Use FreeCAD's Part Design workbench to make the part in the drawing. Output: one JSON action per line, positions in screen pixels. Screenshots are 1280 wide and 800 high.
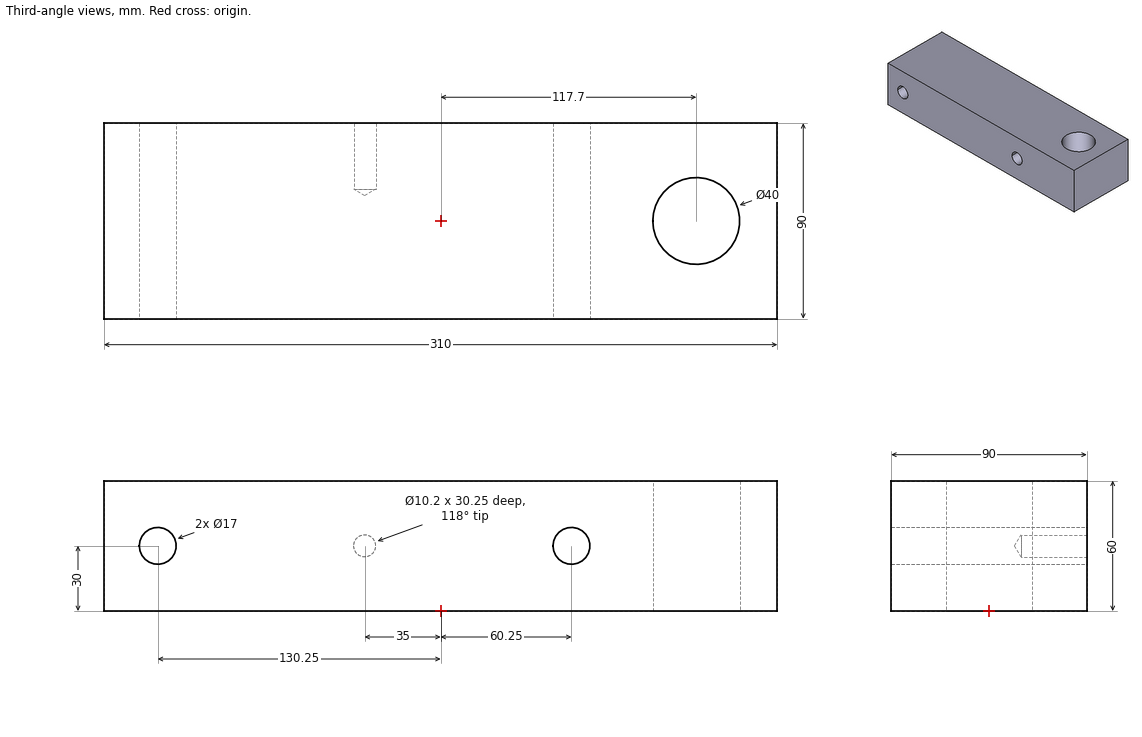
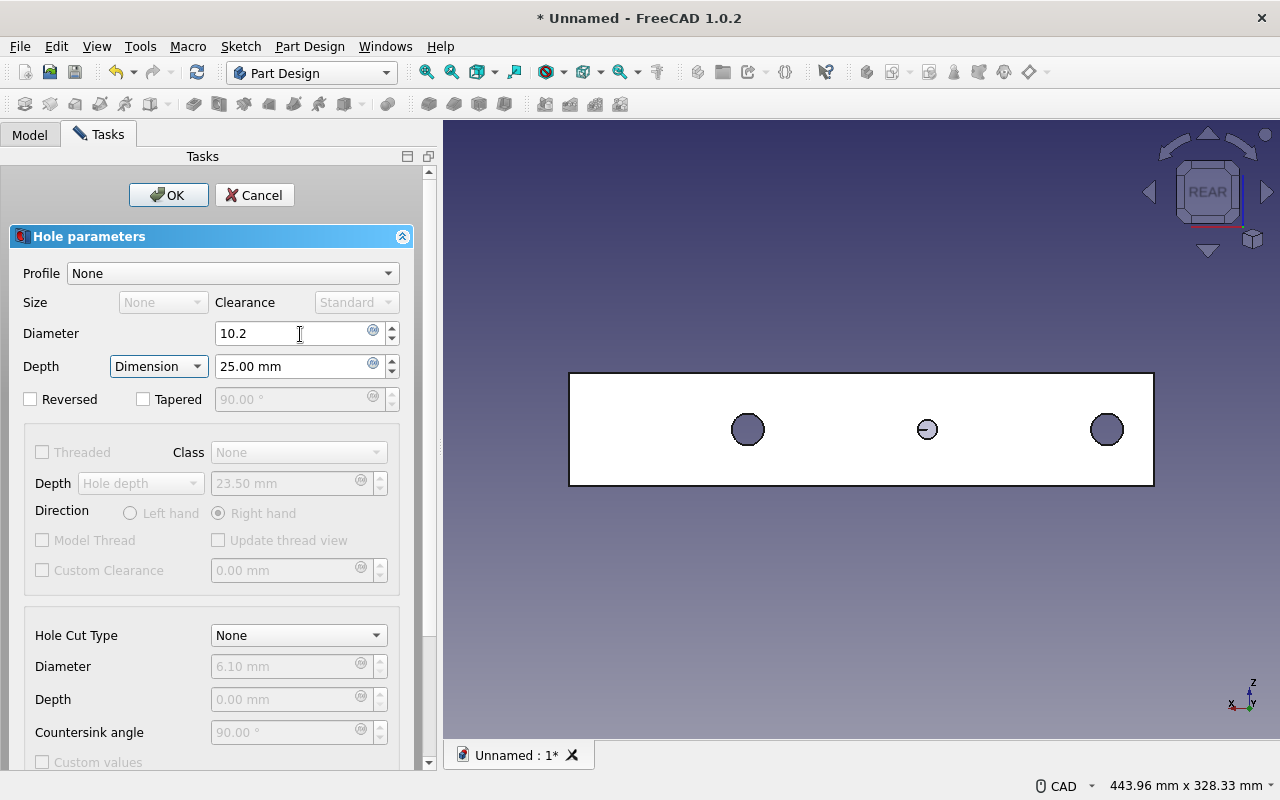
{"action": "triple_click", "coordinate": [300, 366]}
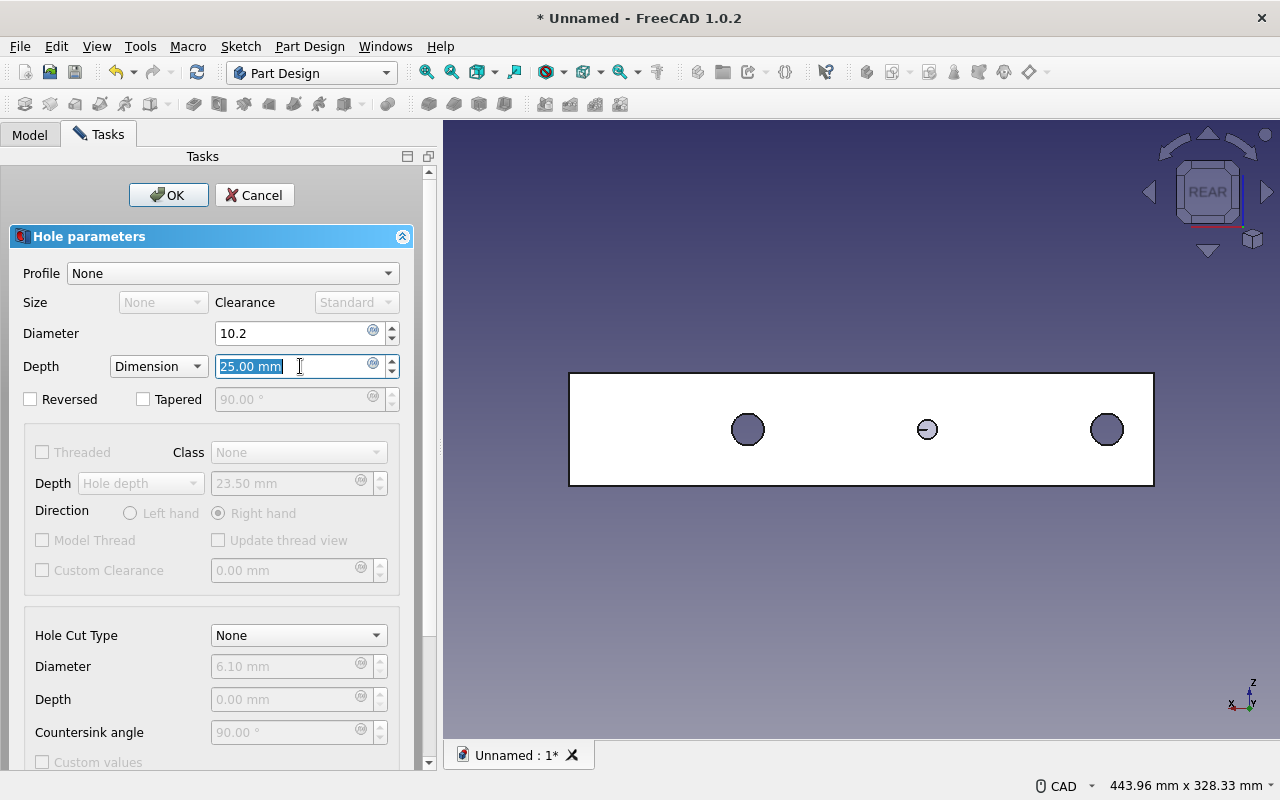
{"action": "type", "text": "30.25"}
{"action": "key", "text": "Tab"}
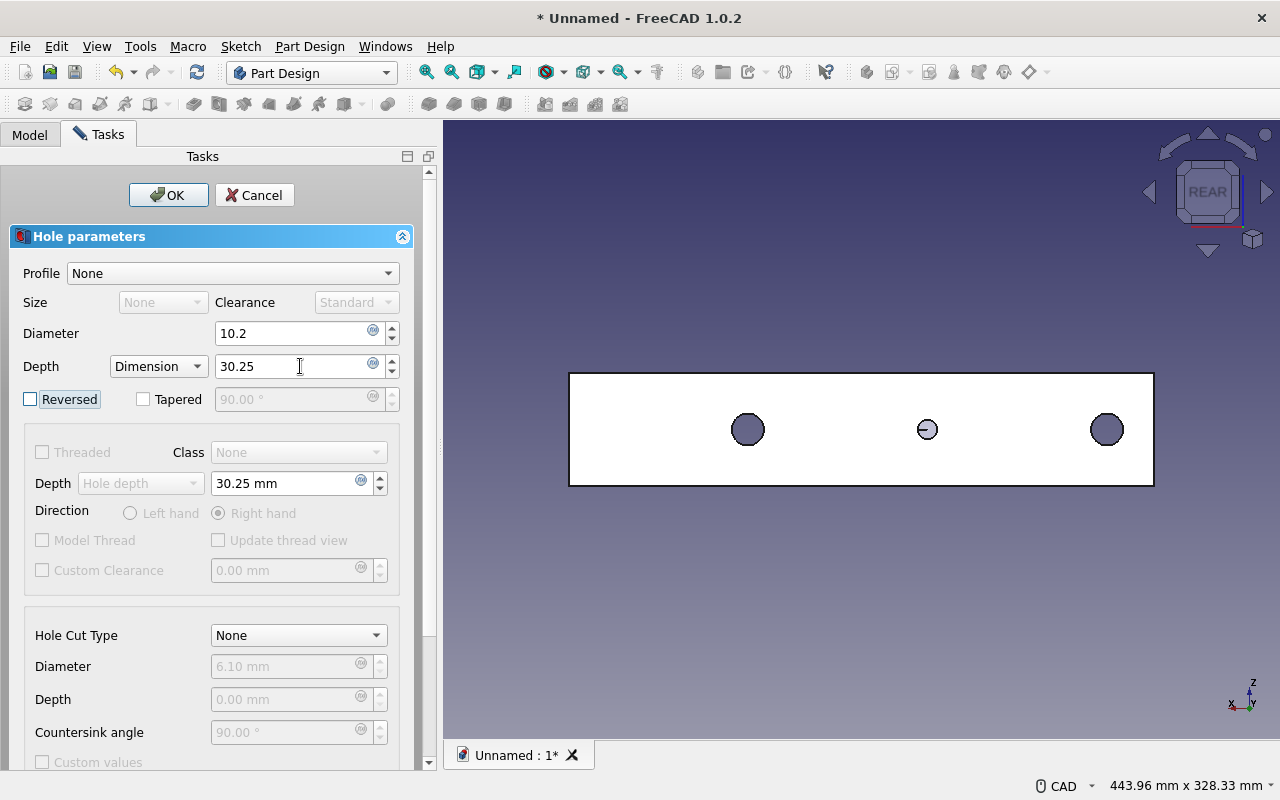
{"action": "left_click", "coordinate": [169, 195]}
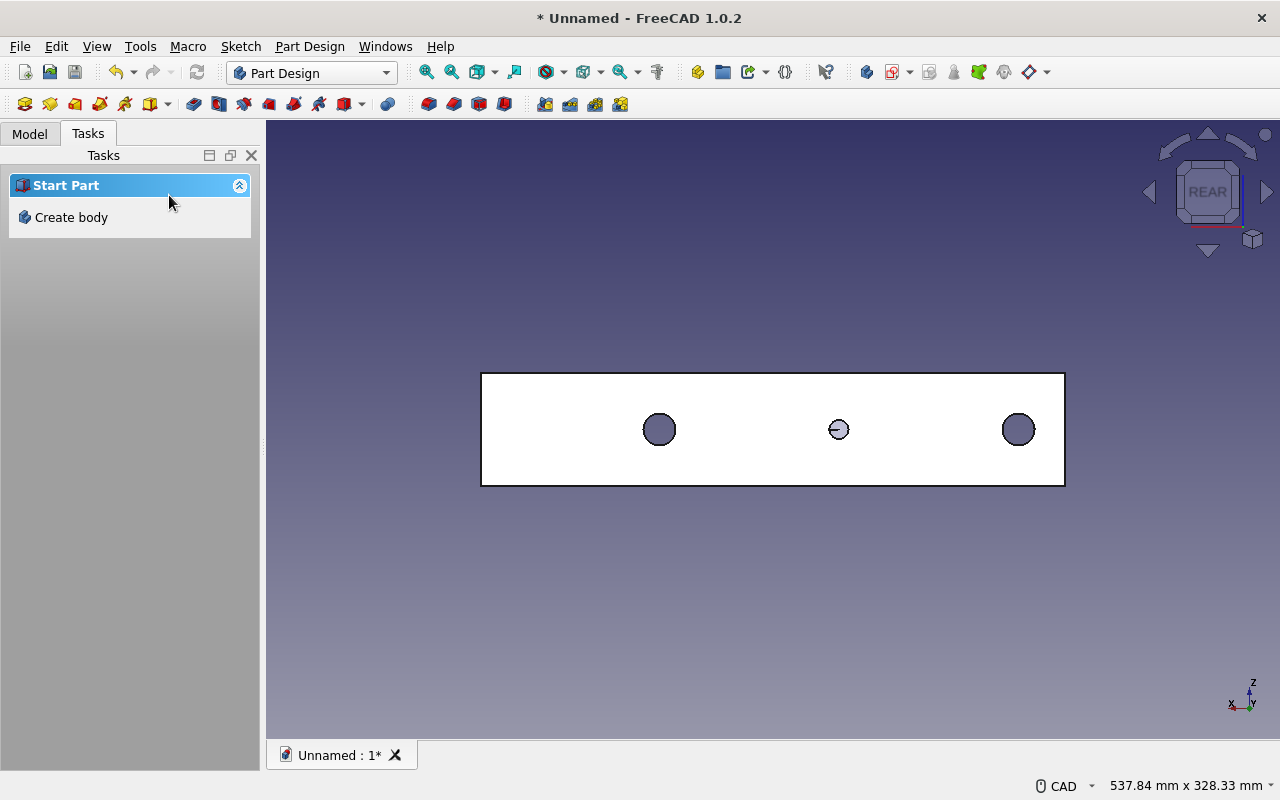
{"action": "left_click", "coordinate": [892, 72]}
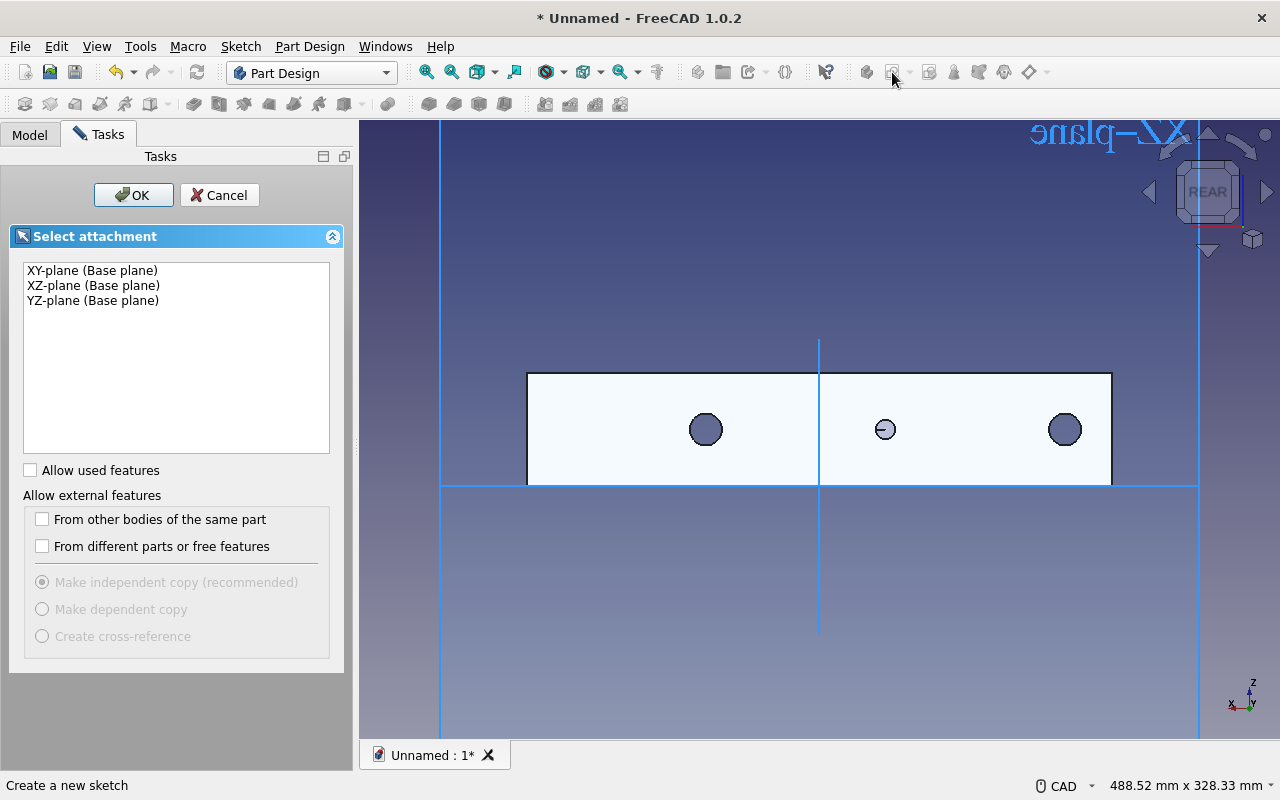
{"action": "left_click", "coordinate": [84, 270]}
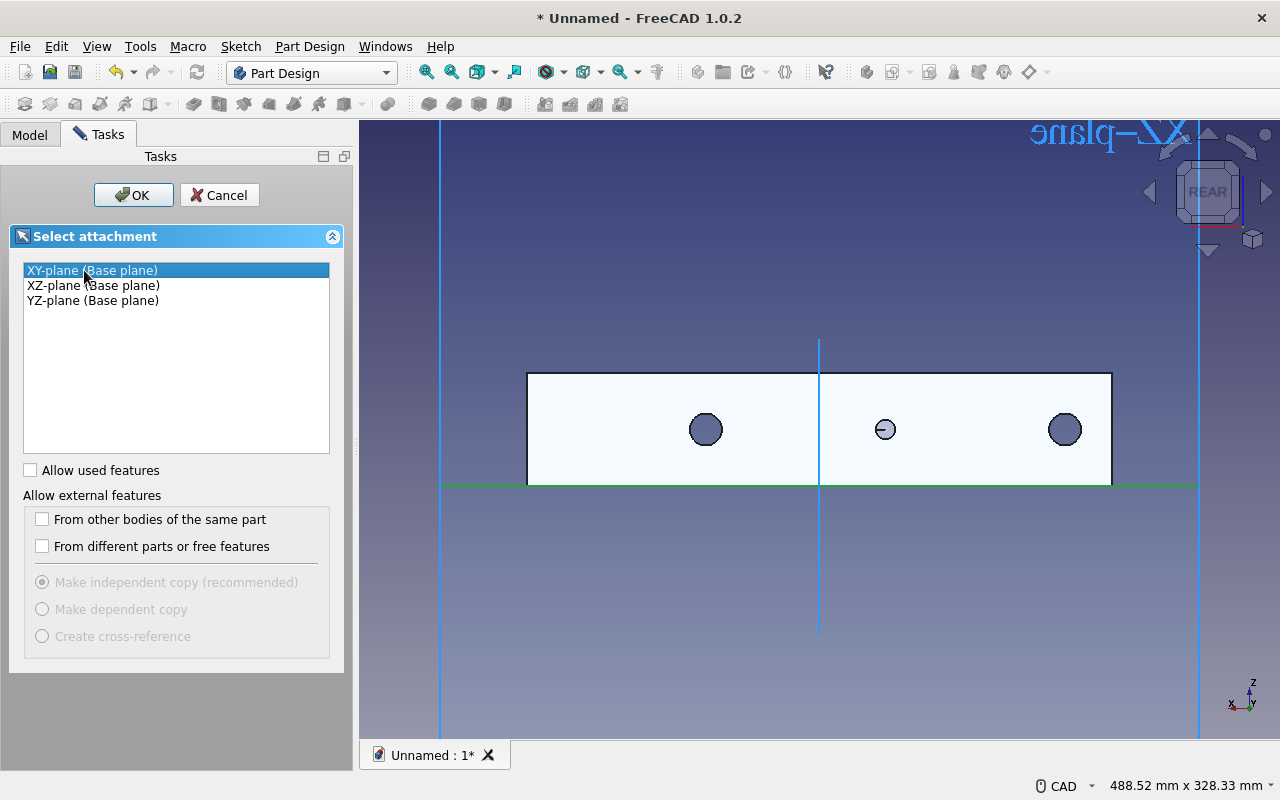
{"action": "left_click", "coordinate": [134, 195]}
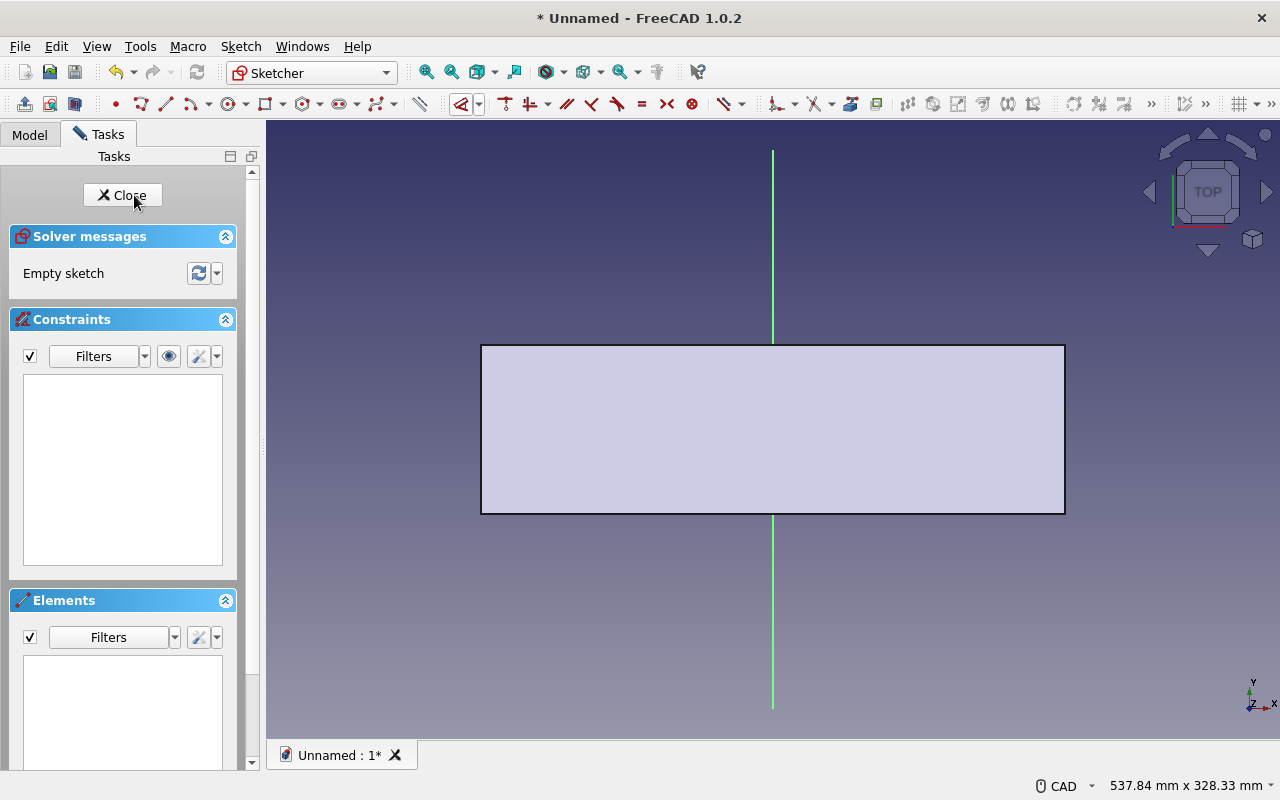
{"action": "left_click", "coordinate": [75, 104]}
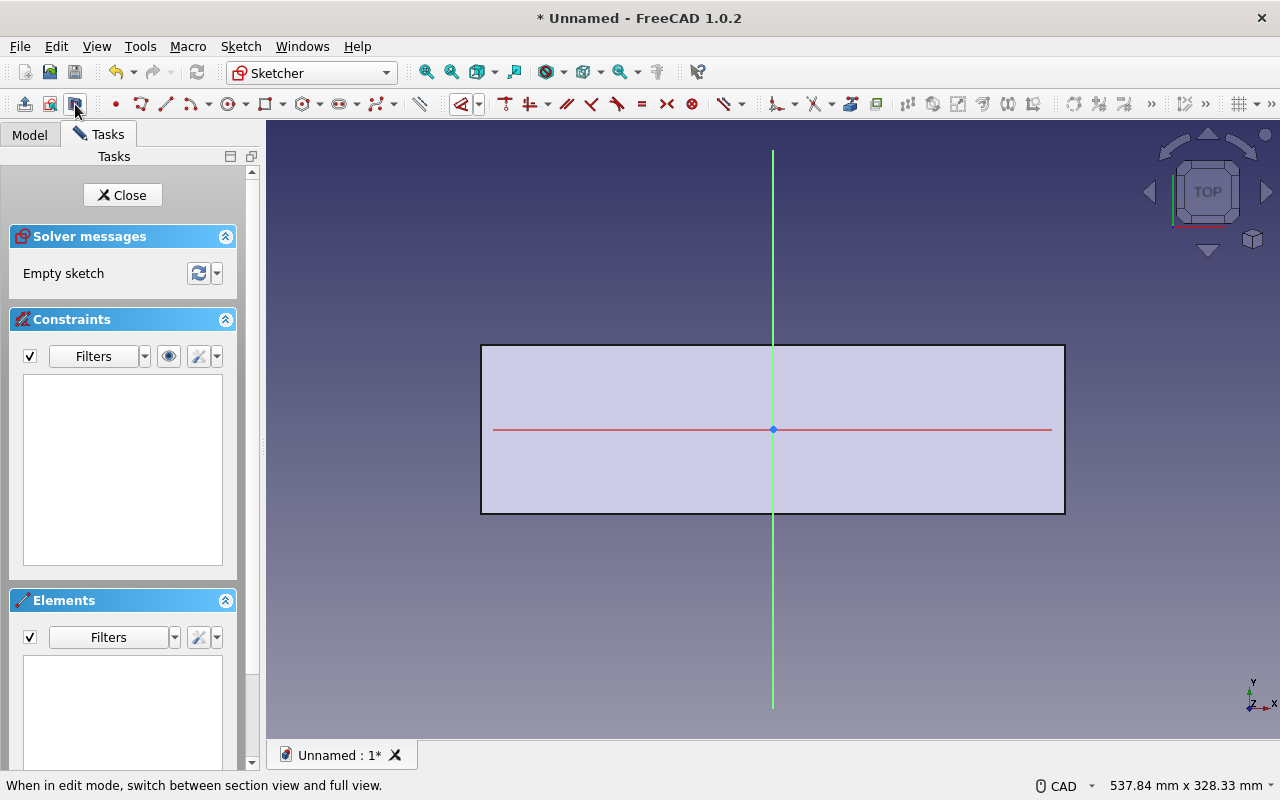
{"action": "scroll", "coordinate": [1068, 429], "scroll_direction": "up", "scroll_amount": 8}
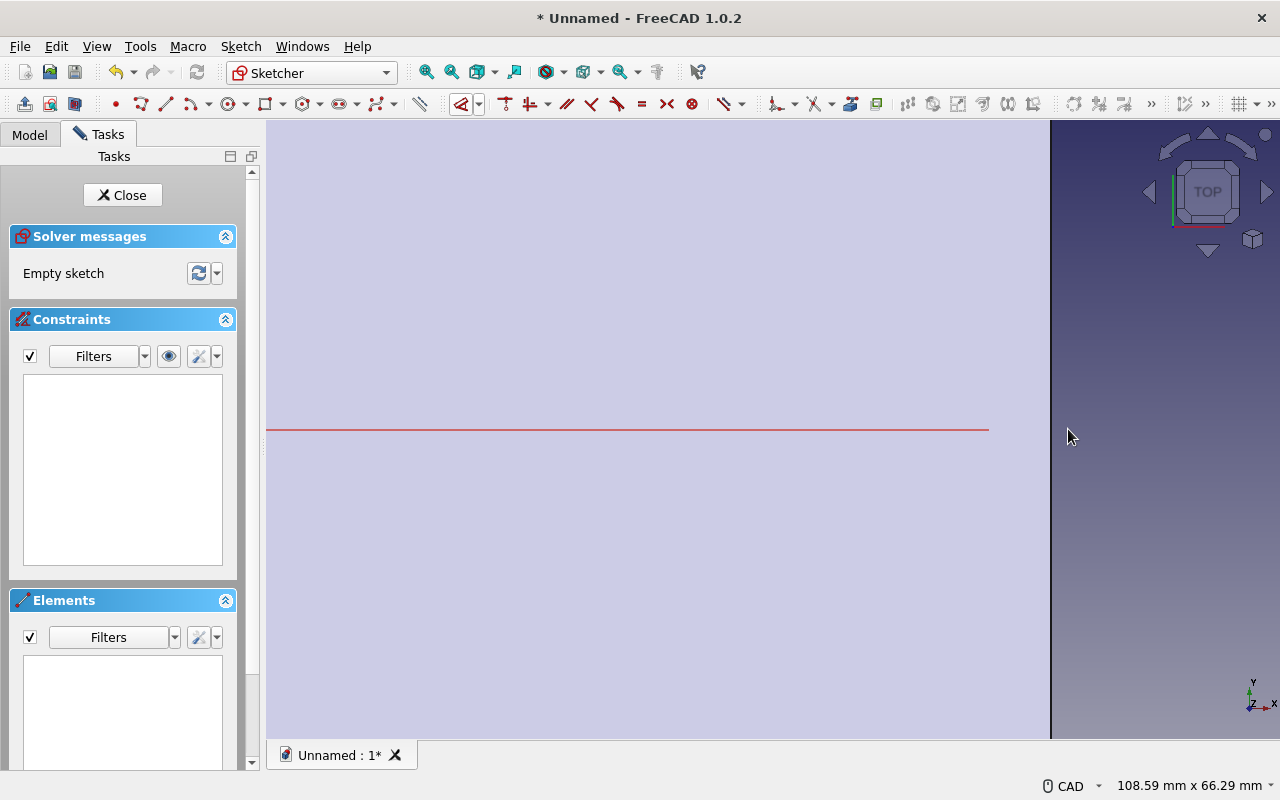
{"action": "key", "text": "g c"}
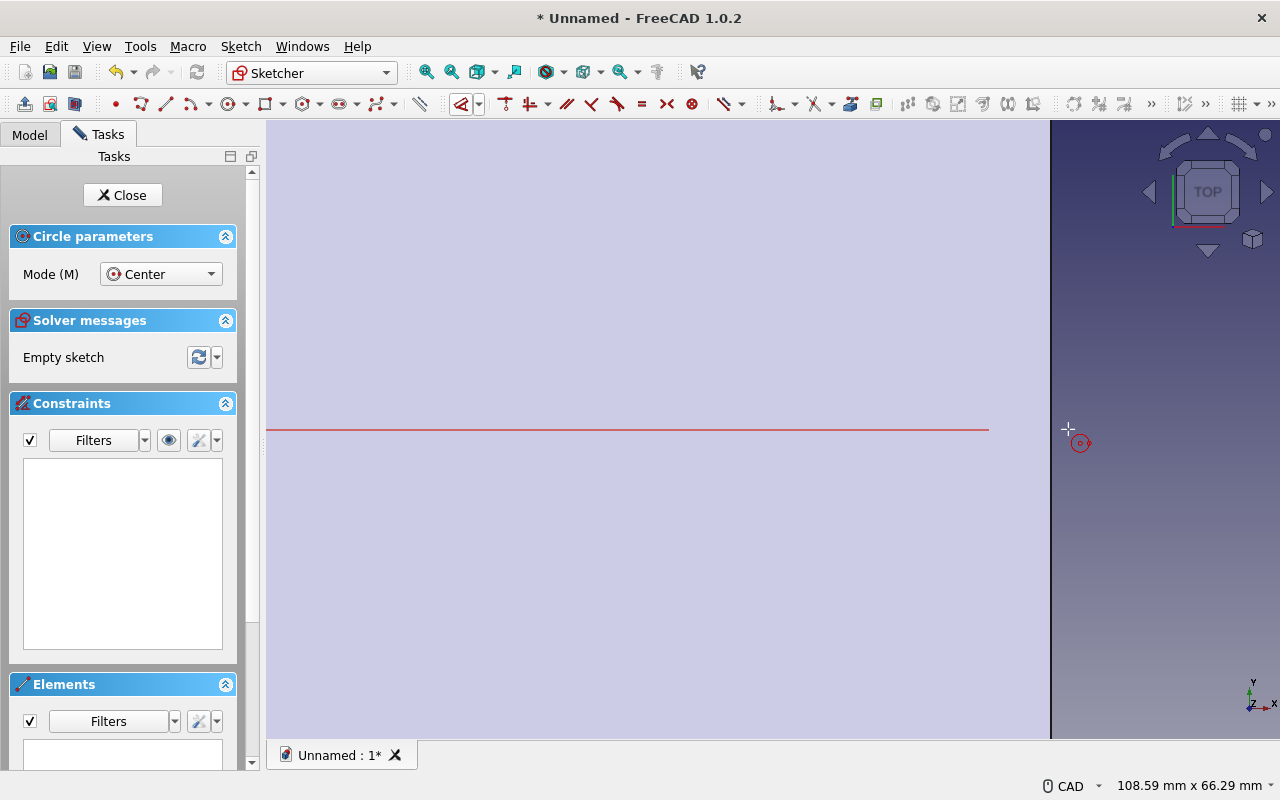
{"action": "left_click", "coordinate": [703, 429]}
{"action": "left_click", "coordinate": [835, 297]}
{"action": "key", "text": "Escape"}